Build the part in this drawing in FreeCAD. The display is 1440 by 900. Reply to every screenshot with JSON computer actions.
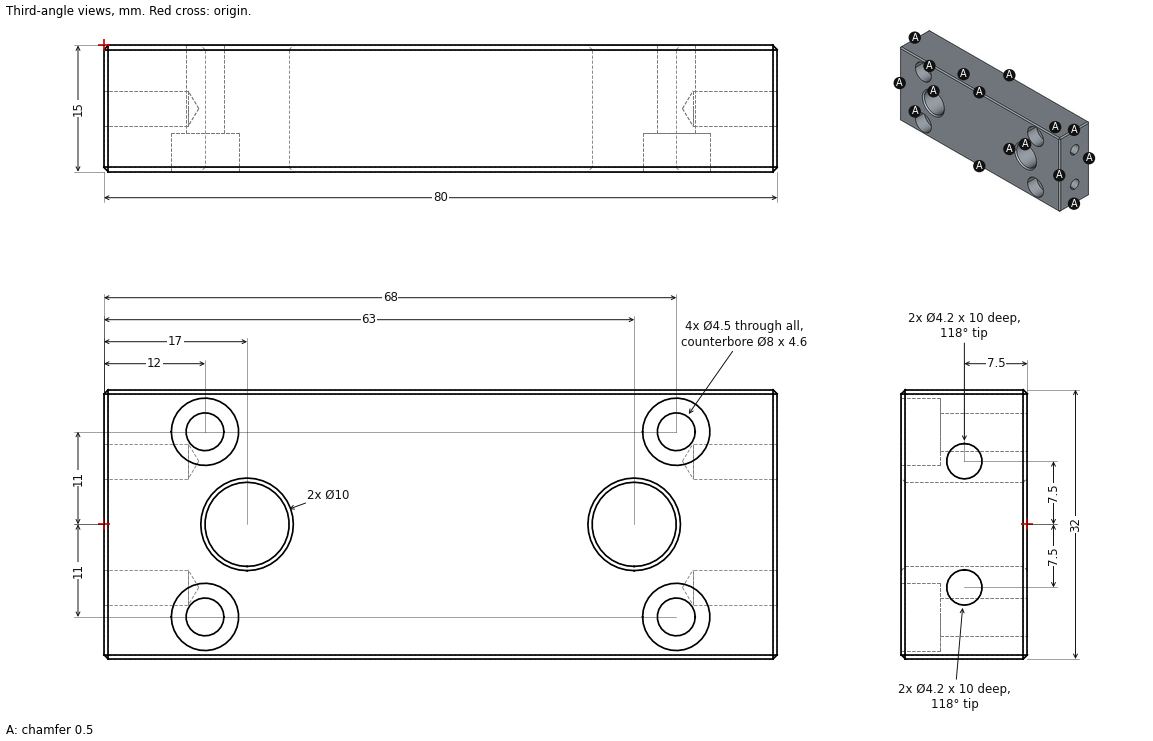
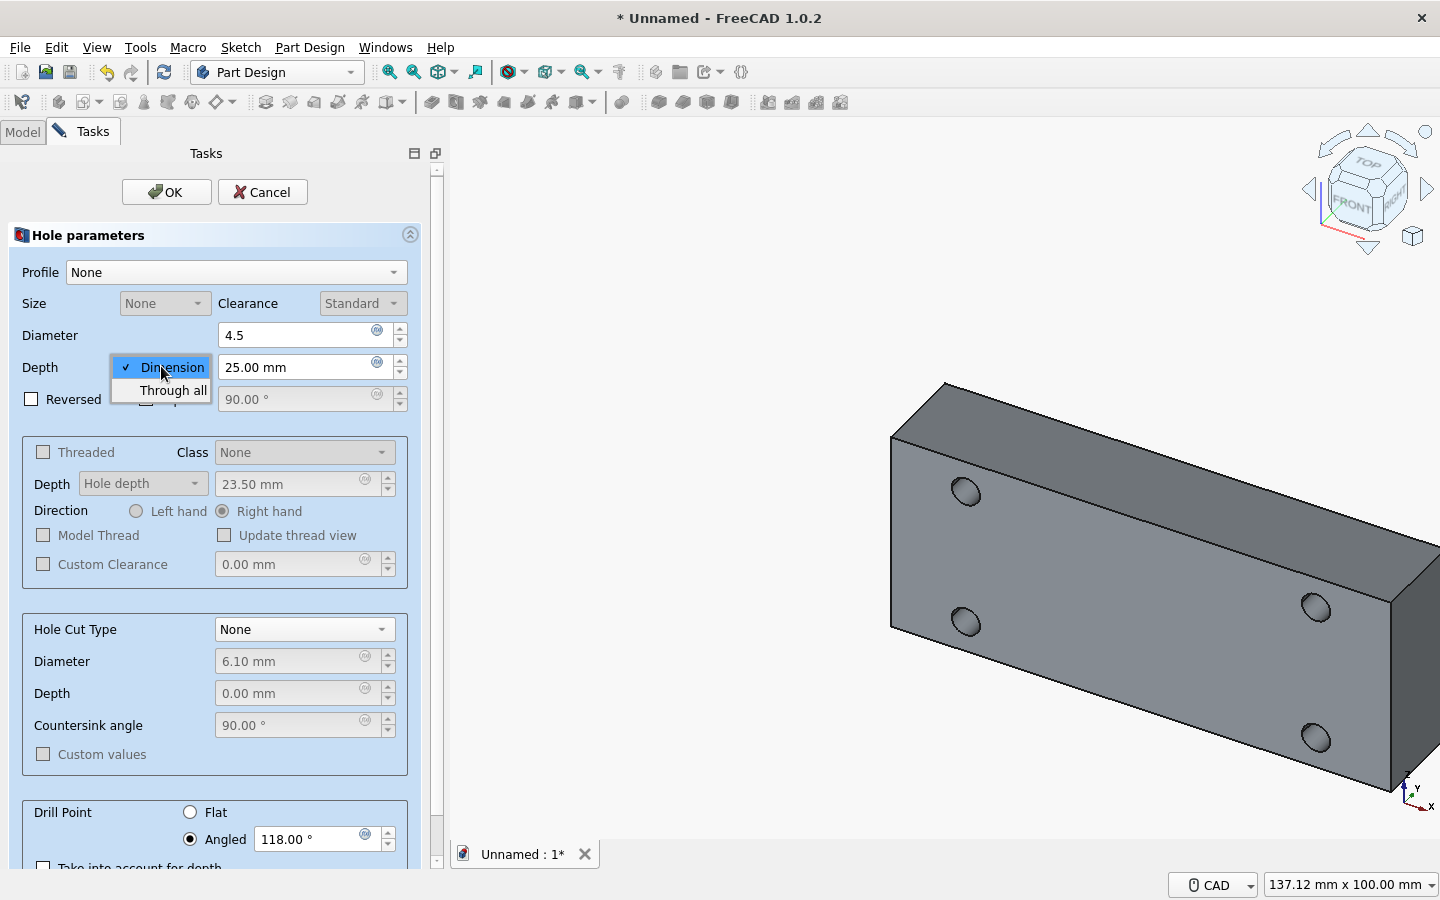
{"action": "left_click", "coordinate": [160, 390]}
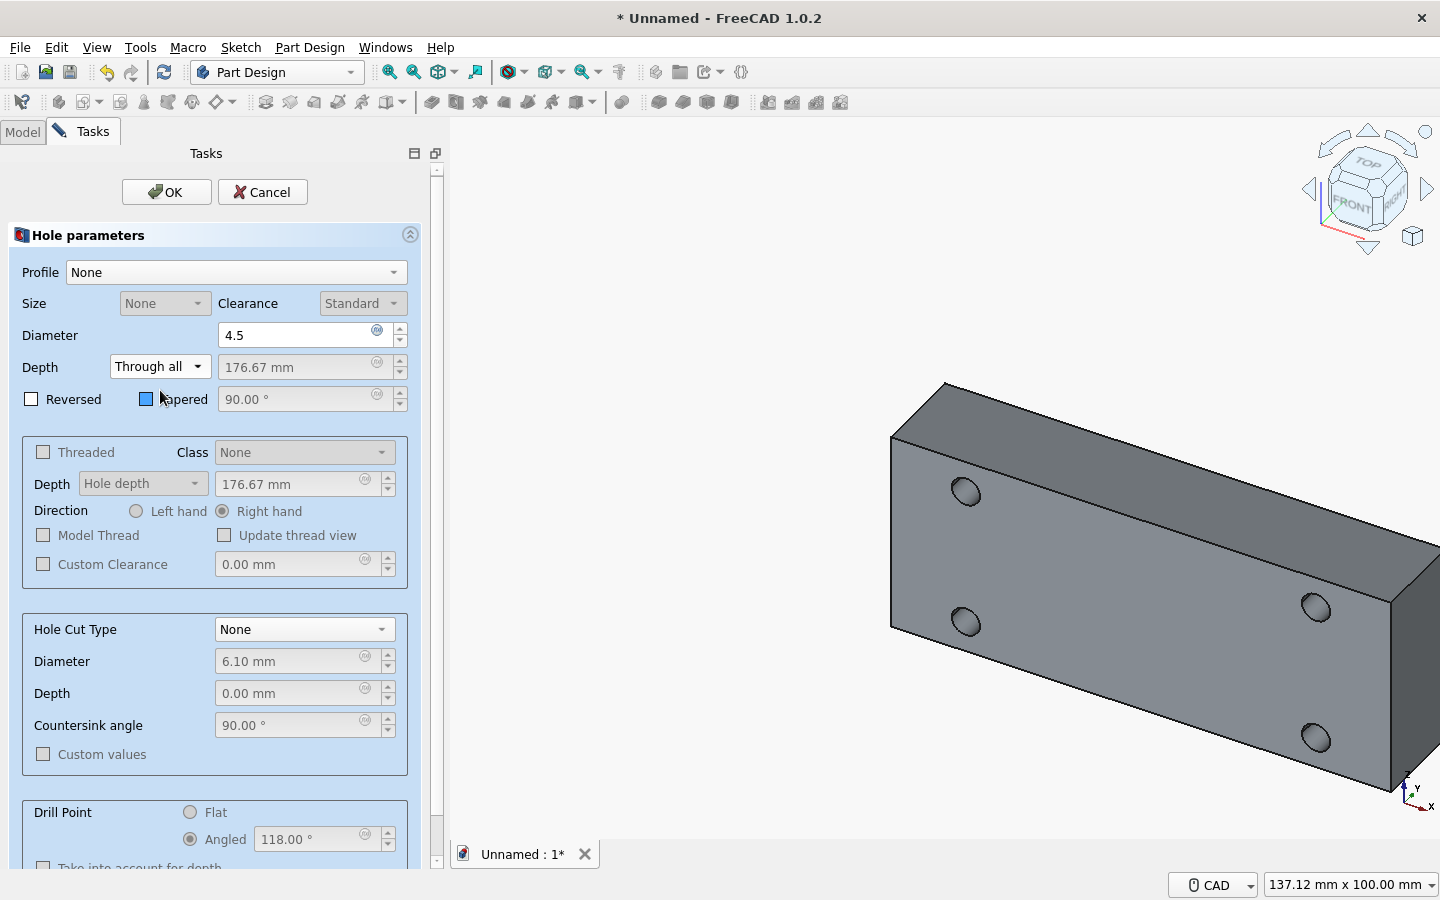
{"action": "left_click", "coordinate": [306, 630]}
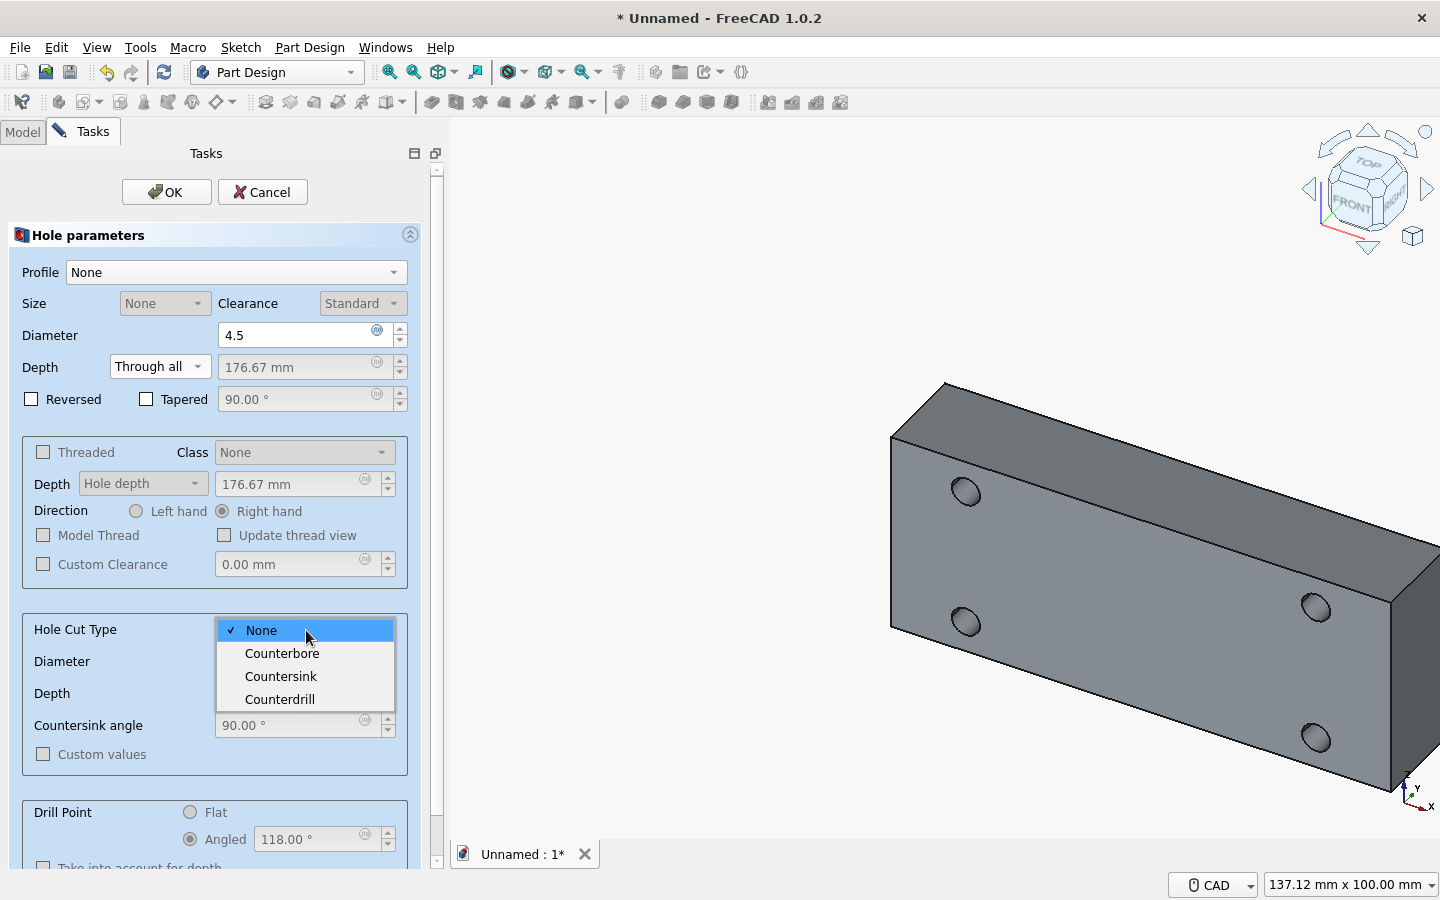
{"action": "left_click", "coordinate": [304, 654]}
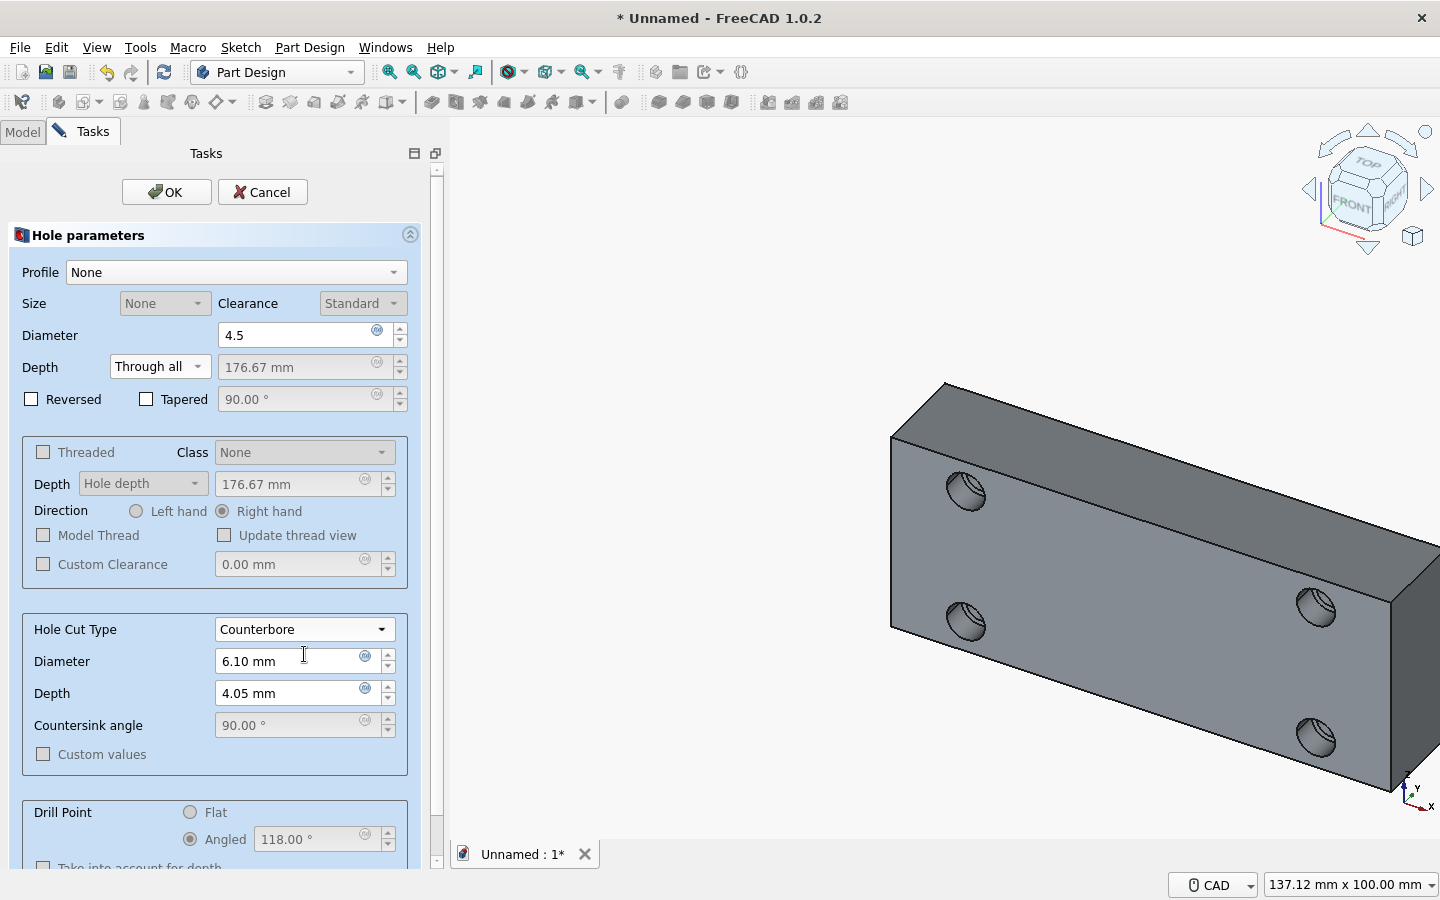
{"action": "triple_click", "coordinate": [298, 661]}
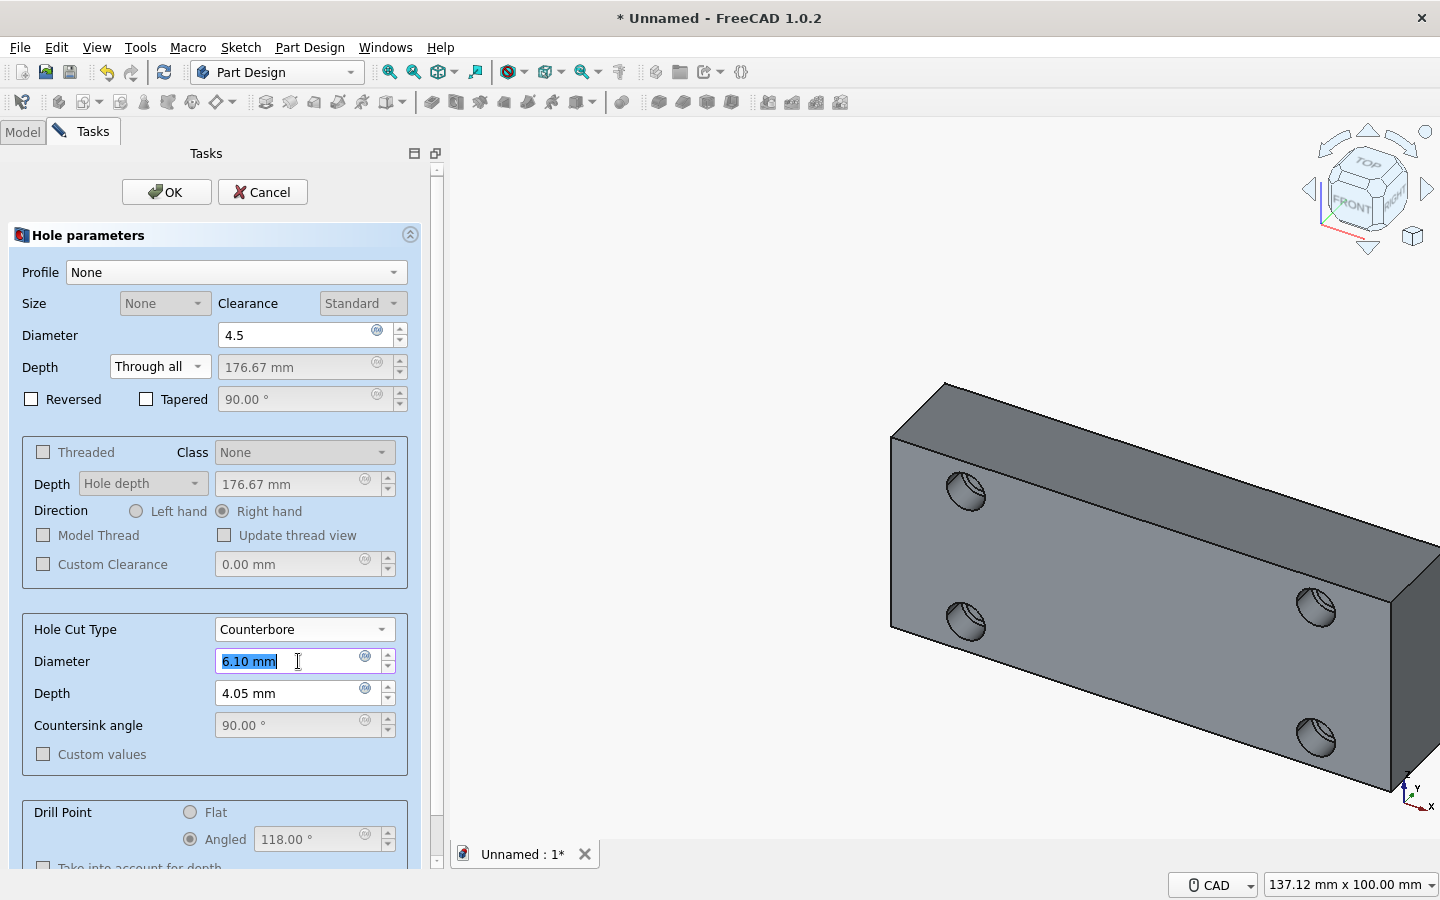
{"action": "type", "text": "8"}
{"action": "key", "text": "Tab"}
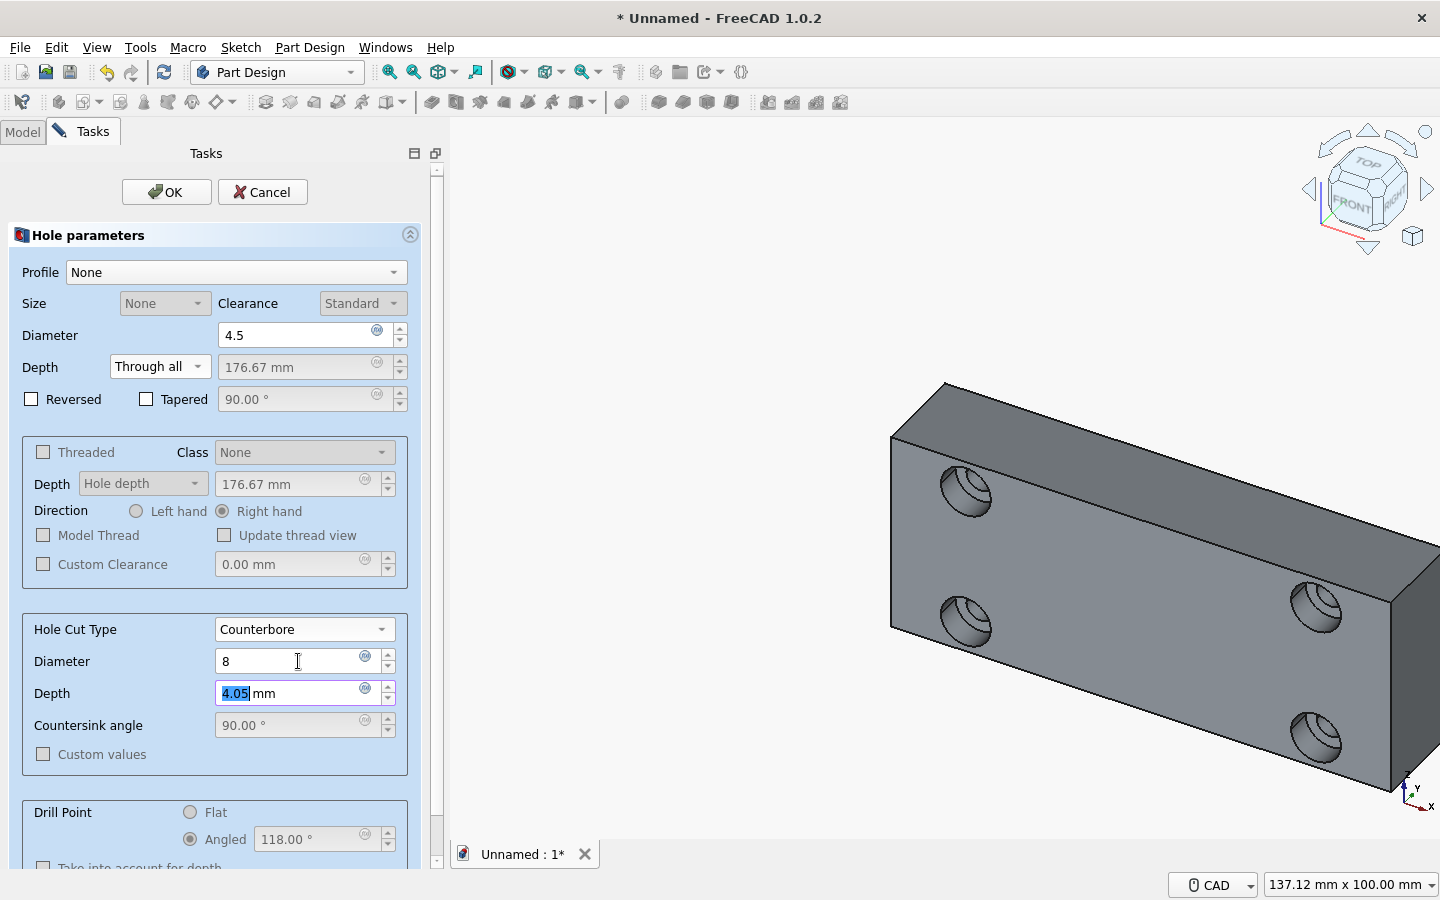
{"action": "type", "text": "4.6"}
{"action": "key", "text": "Tab"}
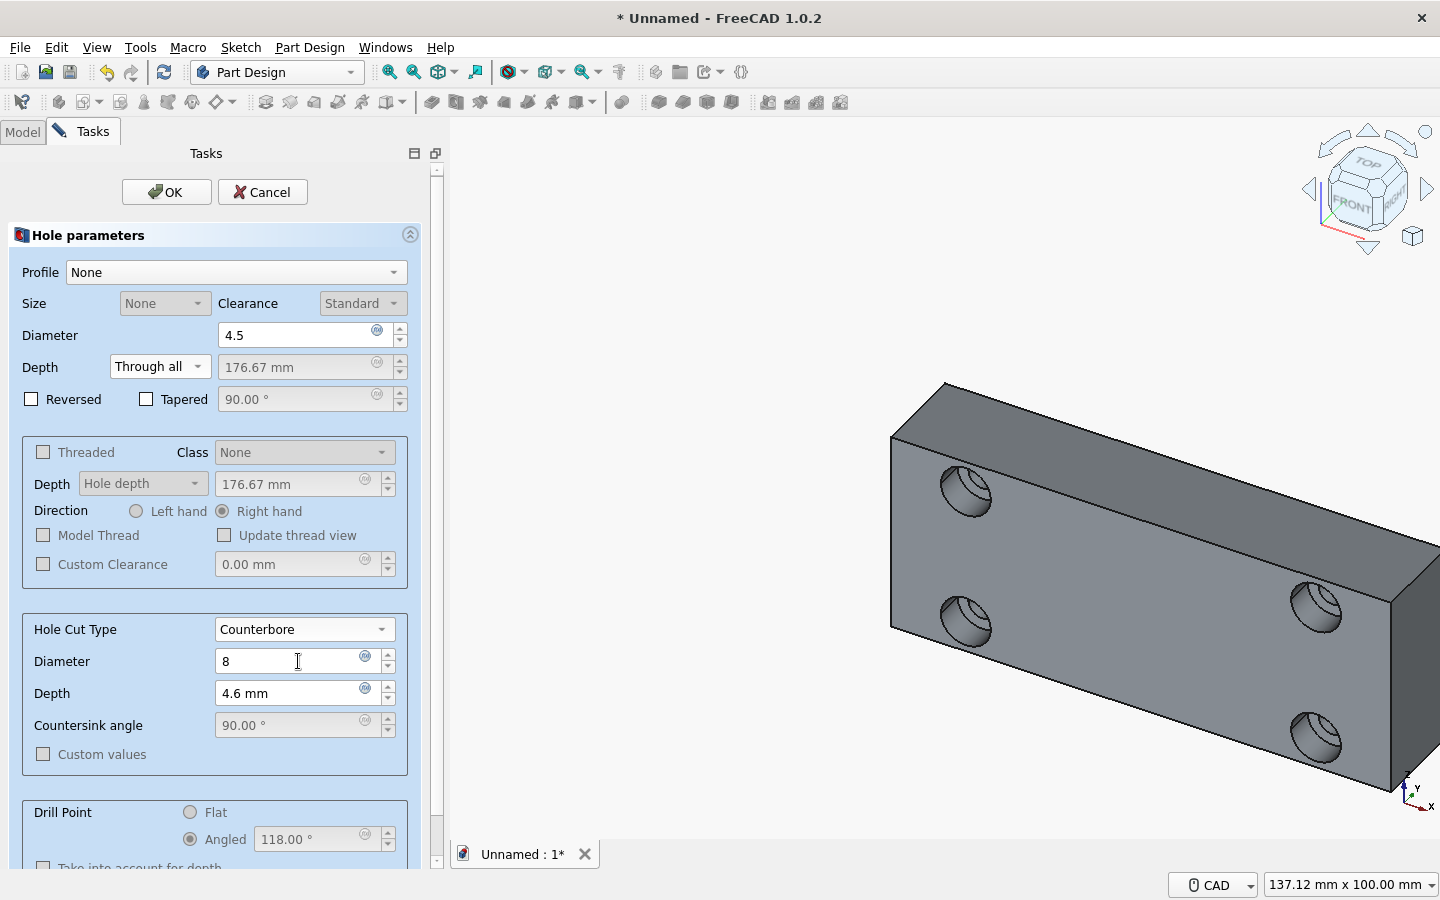
{"action": "left_click", "coordinate": [167, 192]}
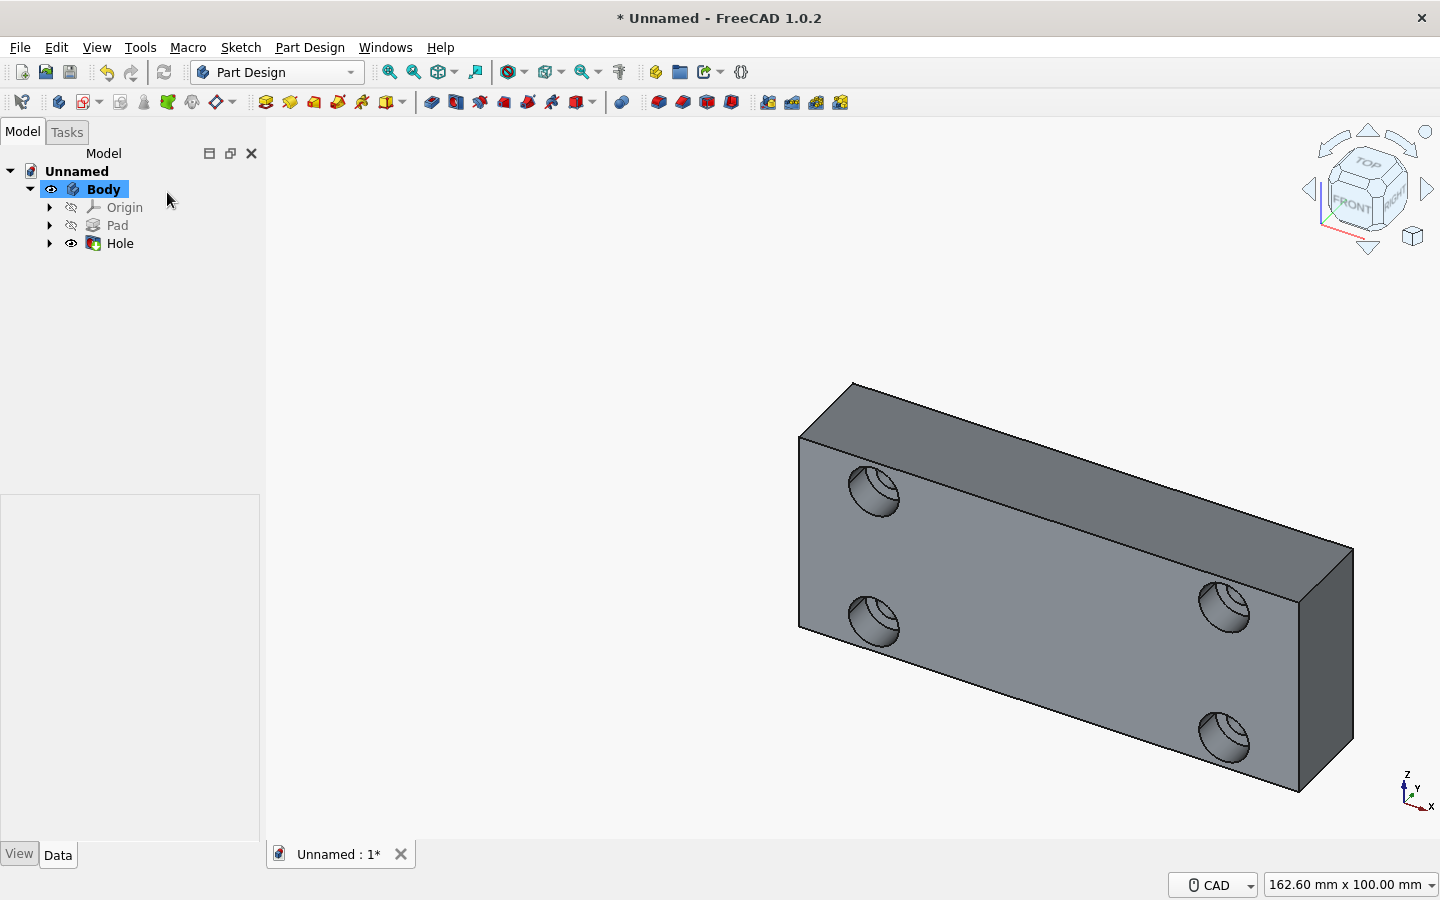
{"action": "left_click", "coordinate": [1049, 614]}